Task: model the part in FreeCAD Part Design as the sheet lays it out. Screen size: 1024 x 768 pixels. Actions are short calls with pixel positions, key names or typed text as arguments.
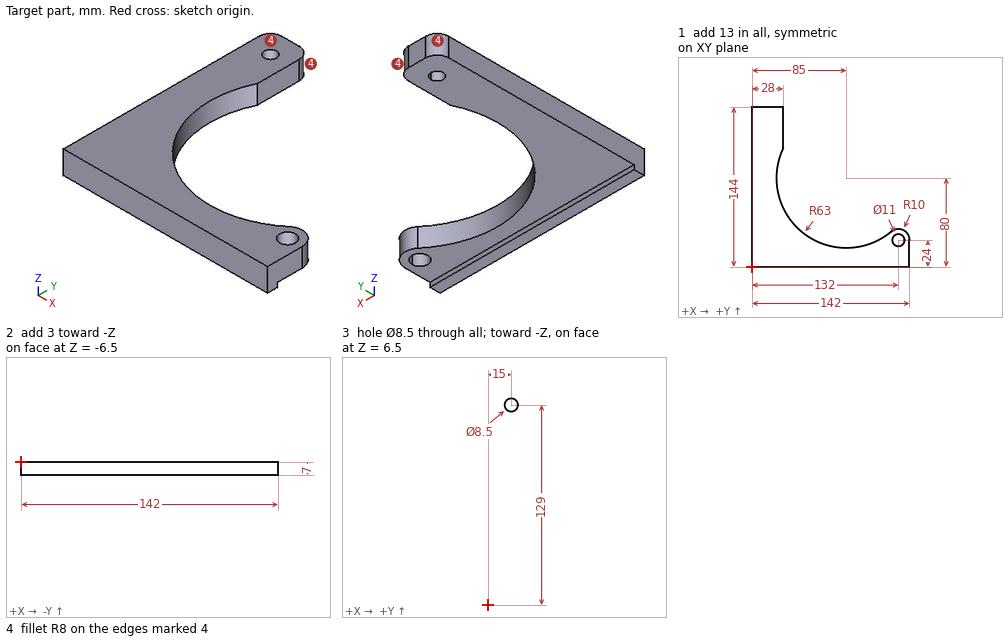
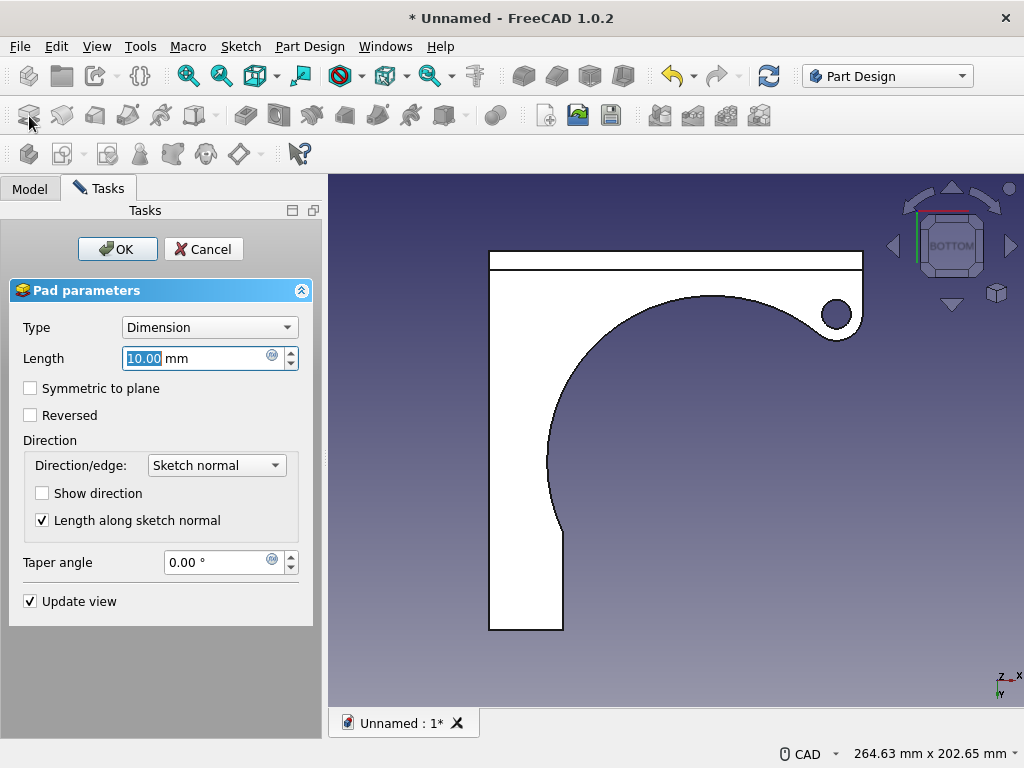
text(3)
key(Tab)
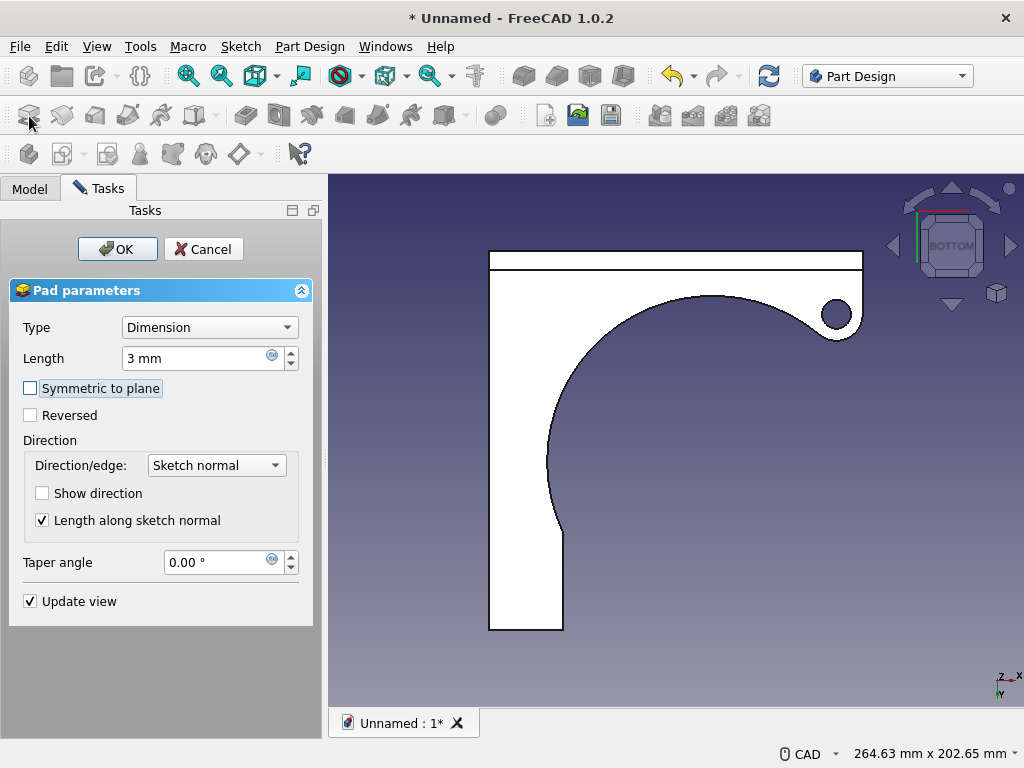
click(118, 249)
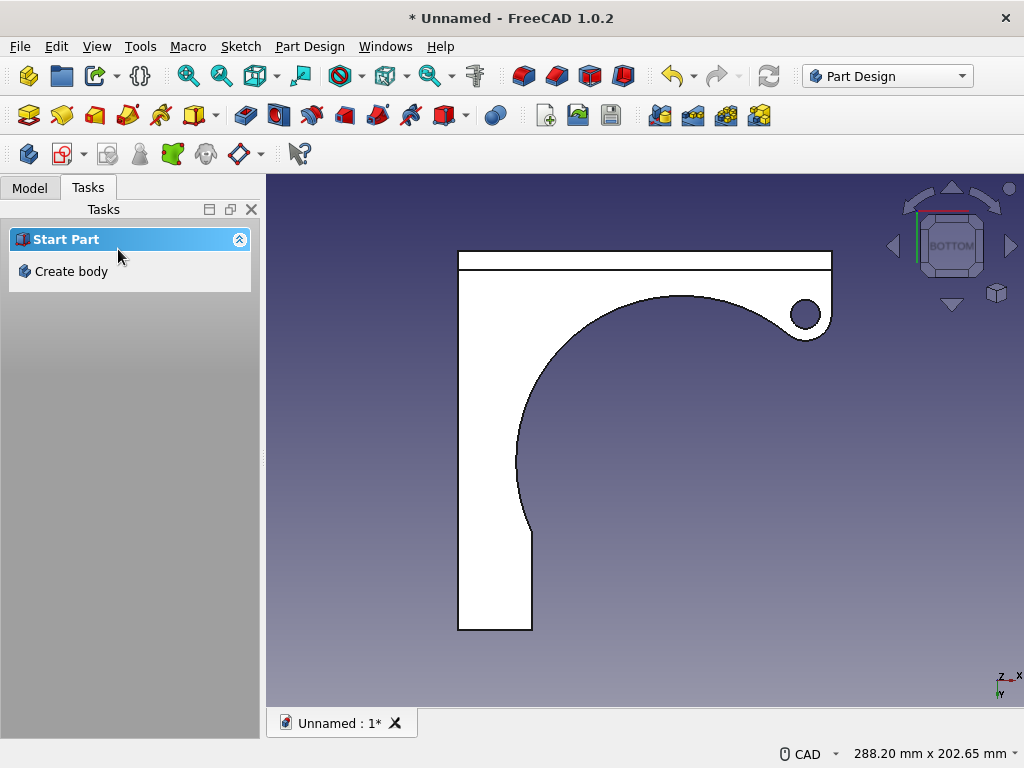
key(0)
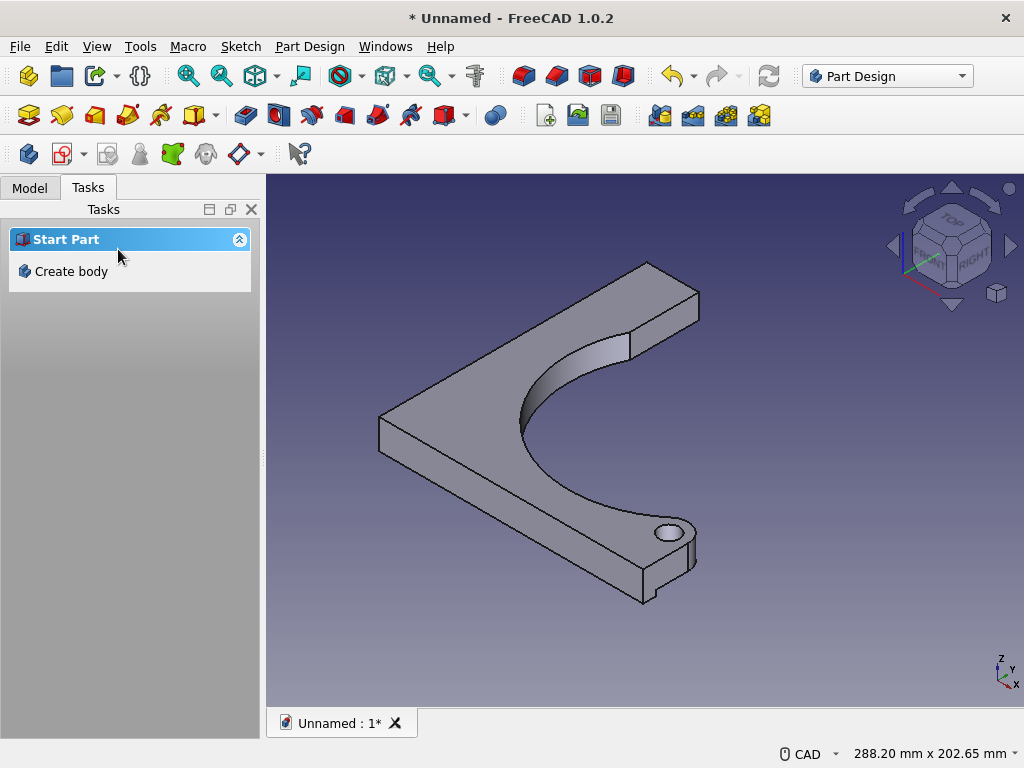
click(493, 415)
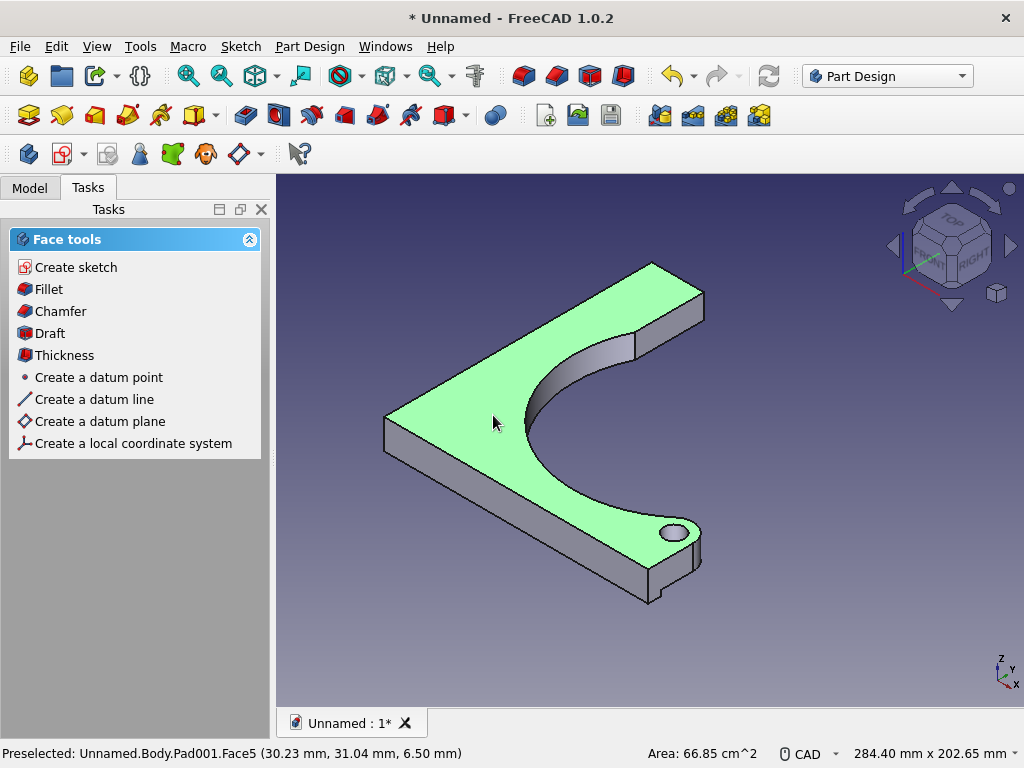
click(62, 154)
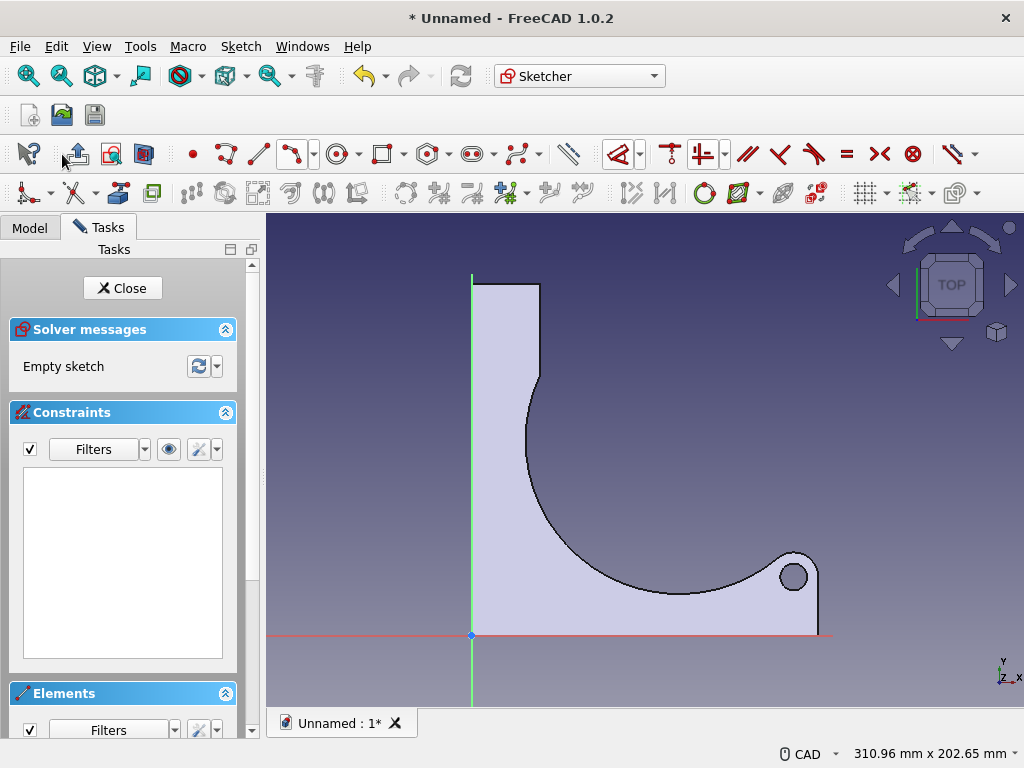
scroll(504, 312, up, 14)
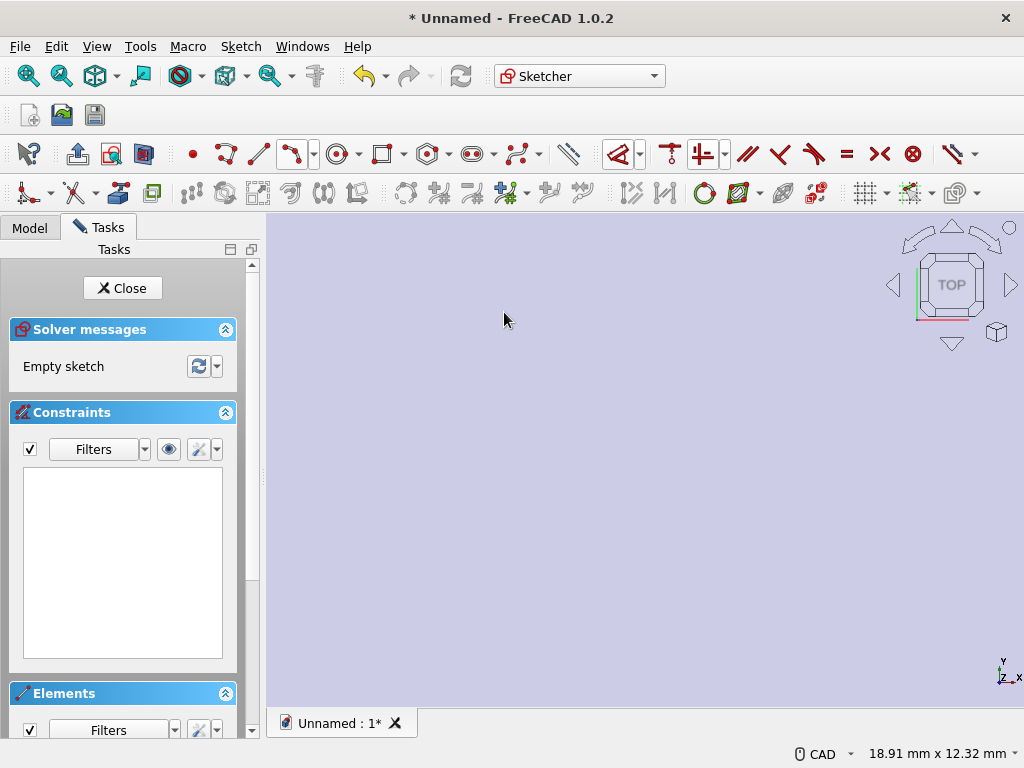
click(336, 154)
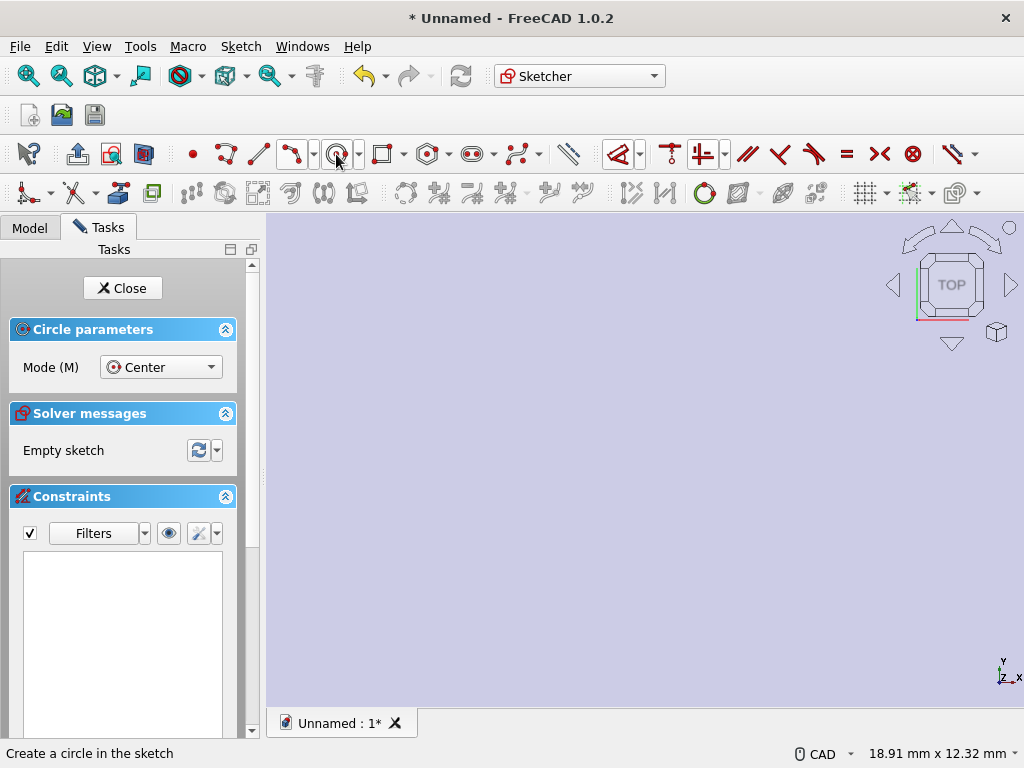
click(573, 458)
move(693, 337)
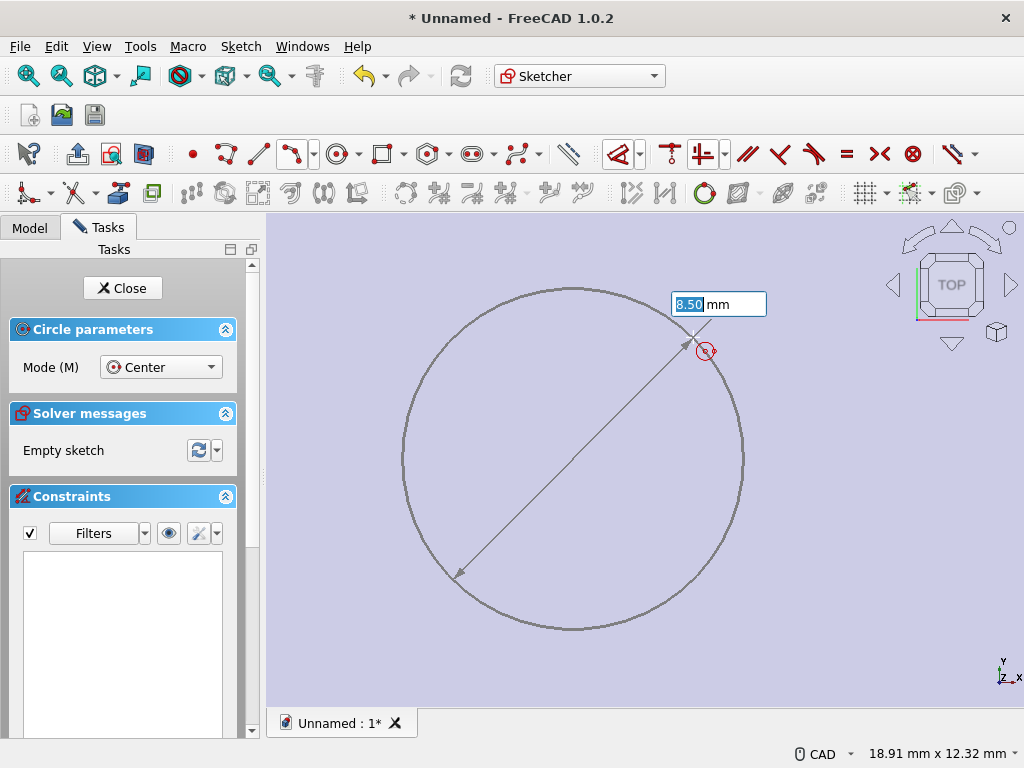
text(8.5)
key(Return)
key(Escape)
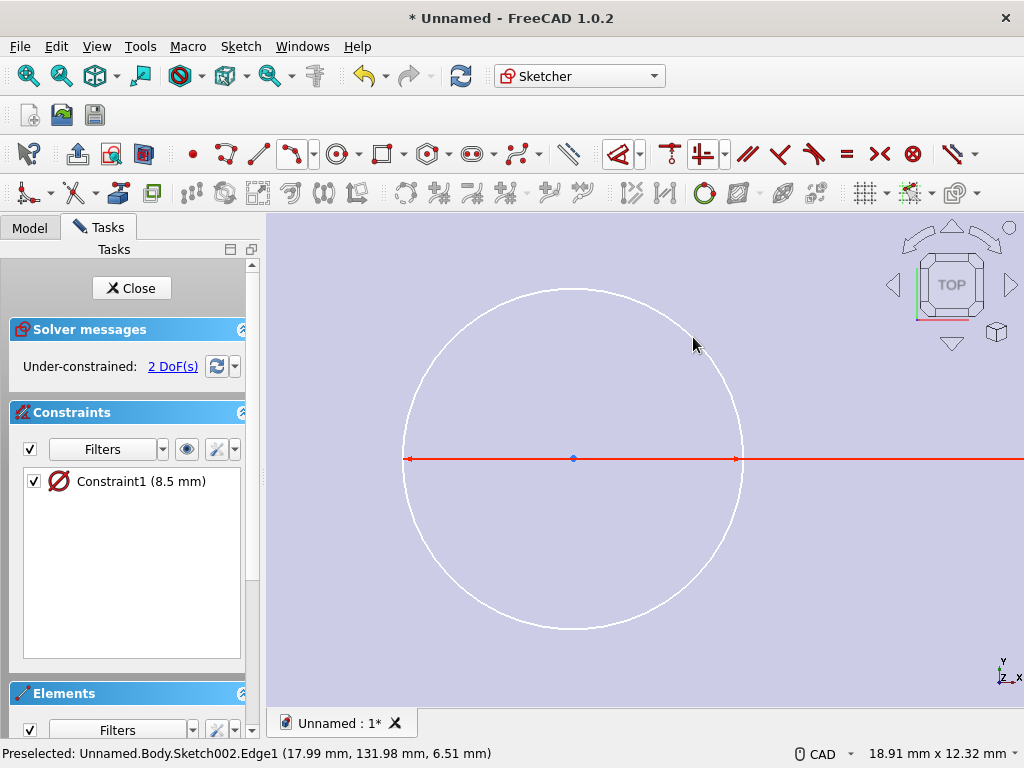
click(573, 459)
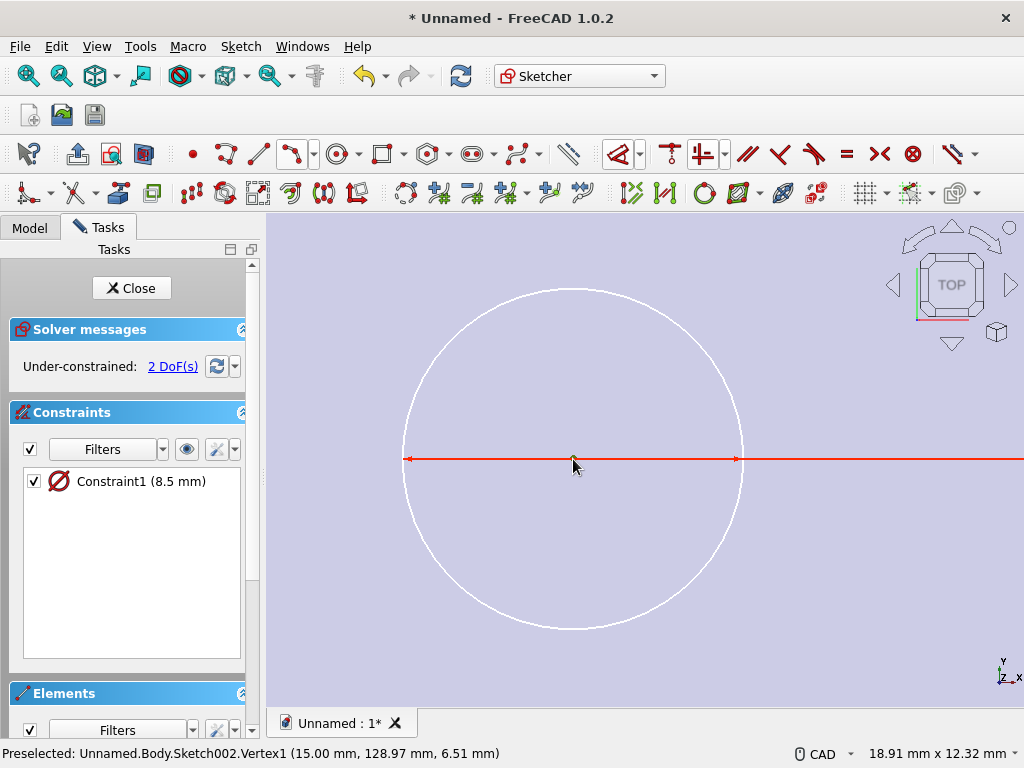
click(640, 154)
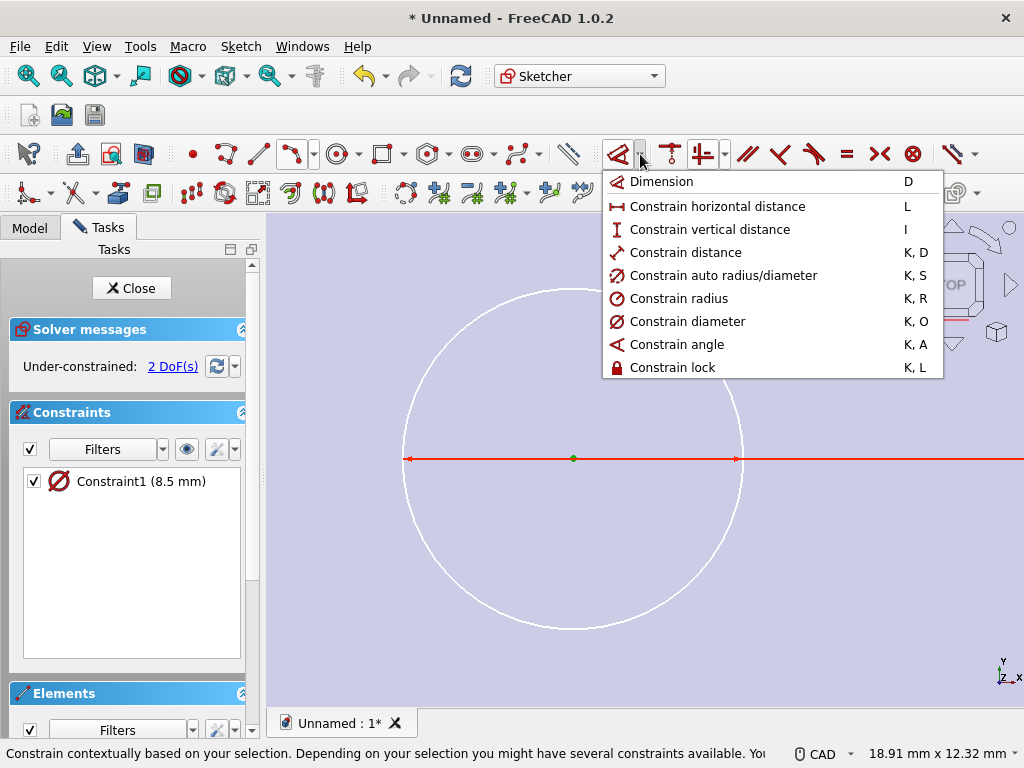
click(773, 206)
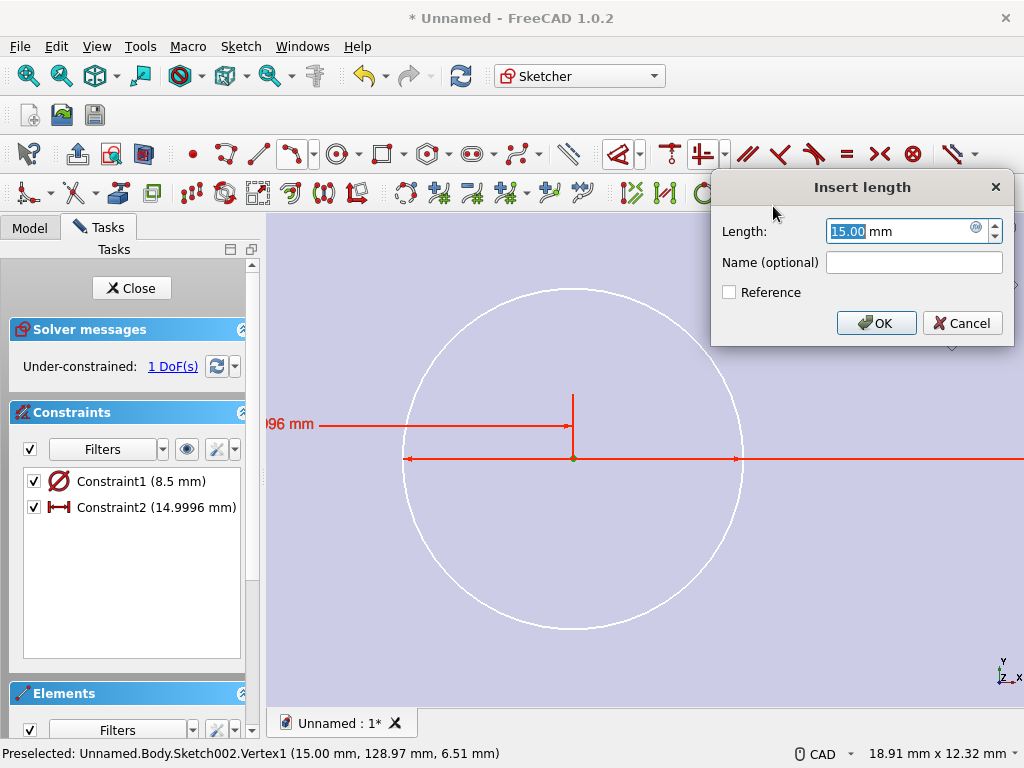
text(15)
key(Return)